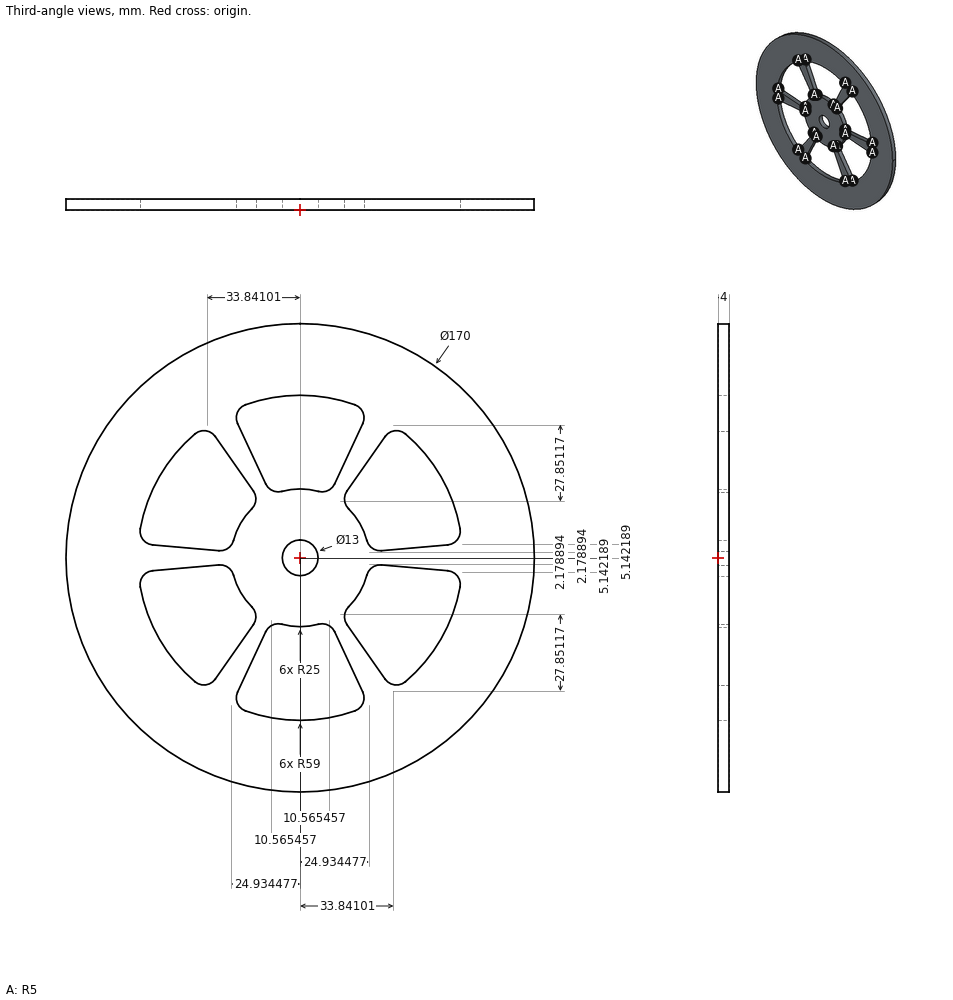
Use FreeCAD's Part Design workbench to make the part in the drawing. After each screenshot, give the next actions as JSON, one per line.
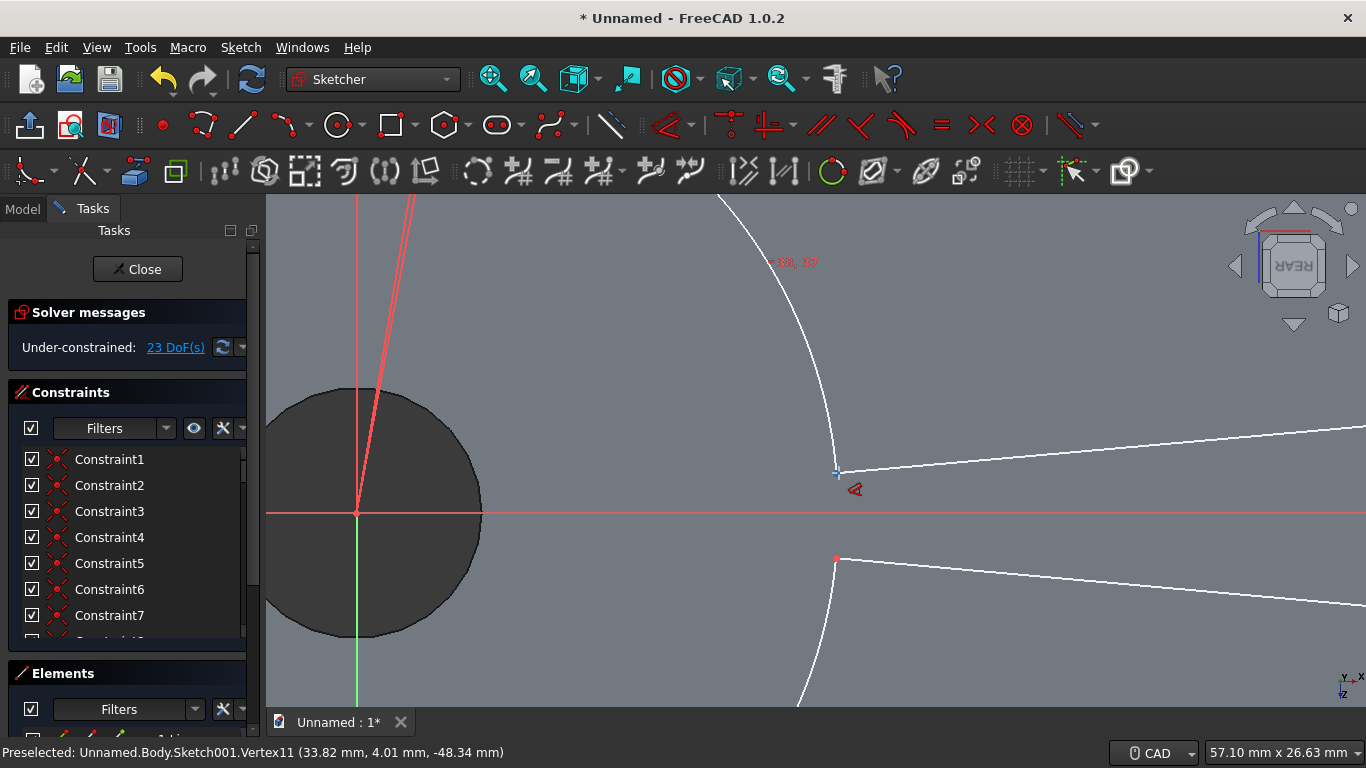
{"action": "left_click", "coordinate": [837, 473]}
{"action": "left_click", "coordinate": [871, 493]}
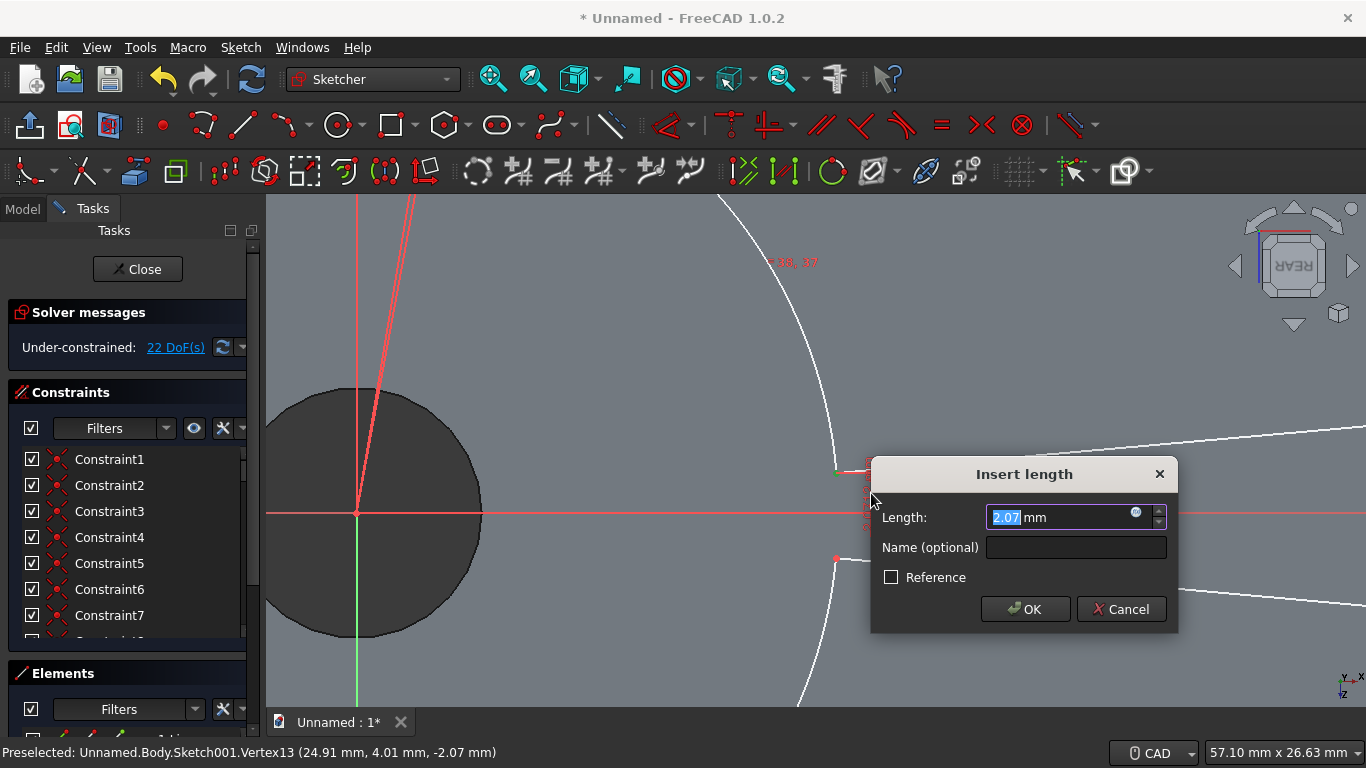
{"action": "type", "text": "2.178894"}
{"action": "key", "text": "Return"}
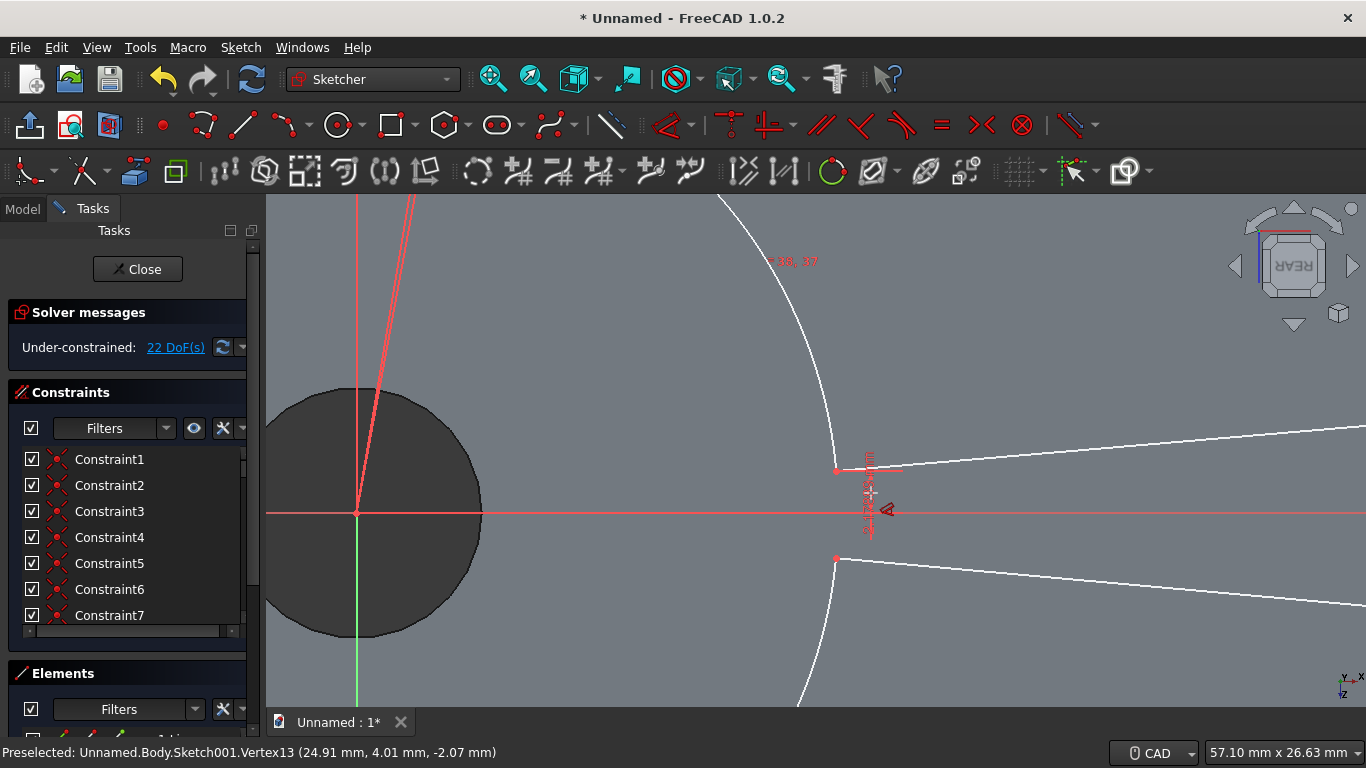
{"action": "scroll", "coordinate": [809, 441], "scroll_direction": "down", "scroll_amount": 10}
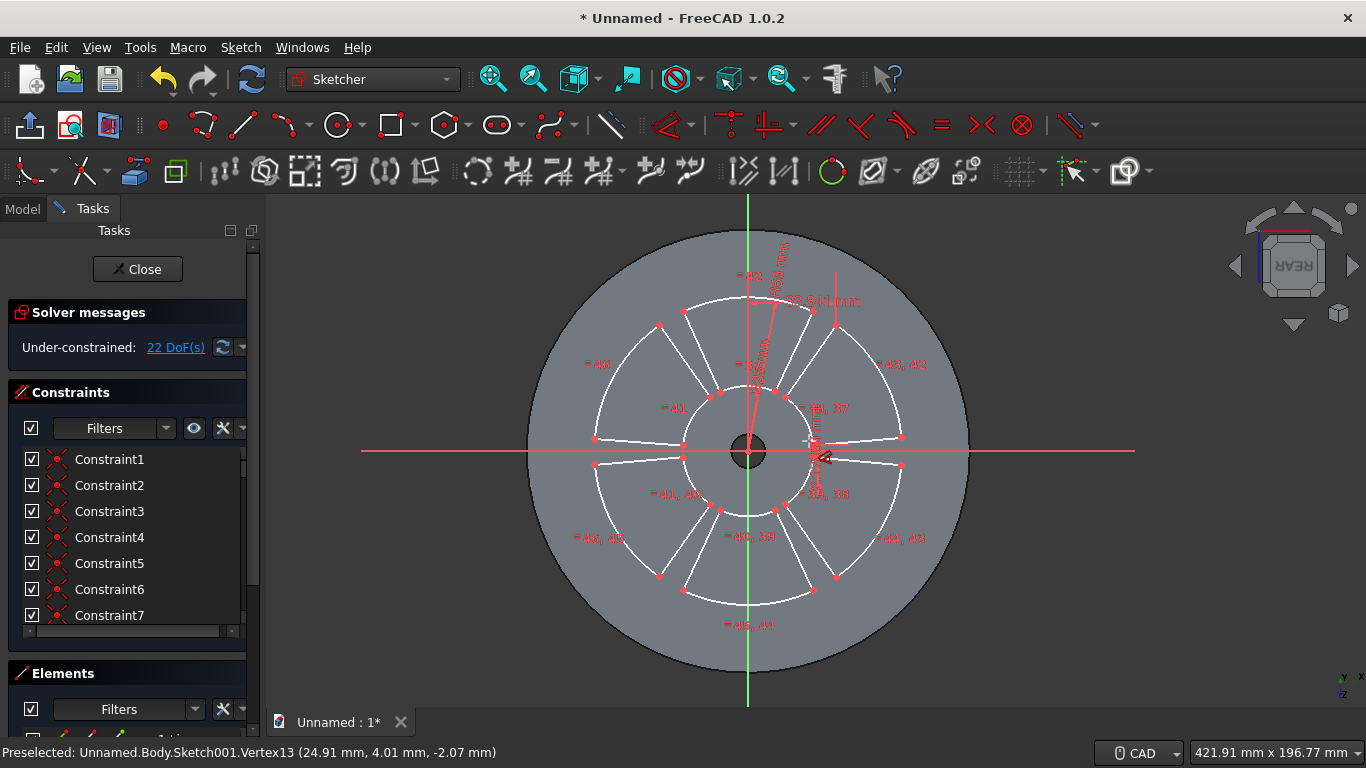
{"action": "scroll", "coordinate": [901, 438], "scroll_direction": "up", "scroll_amount": 6}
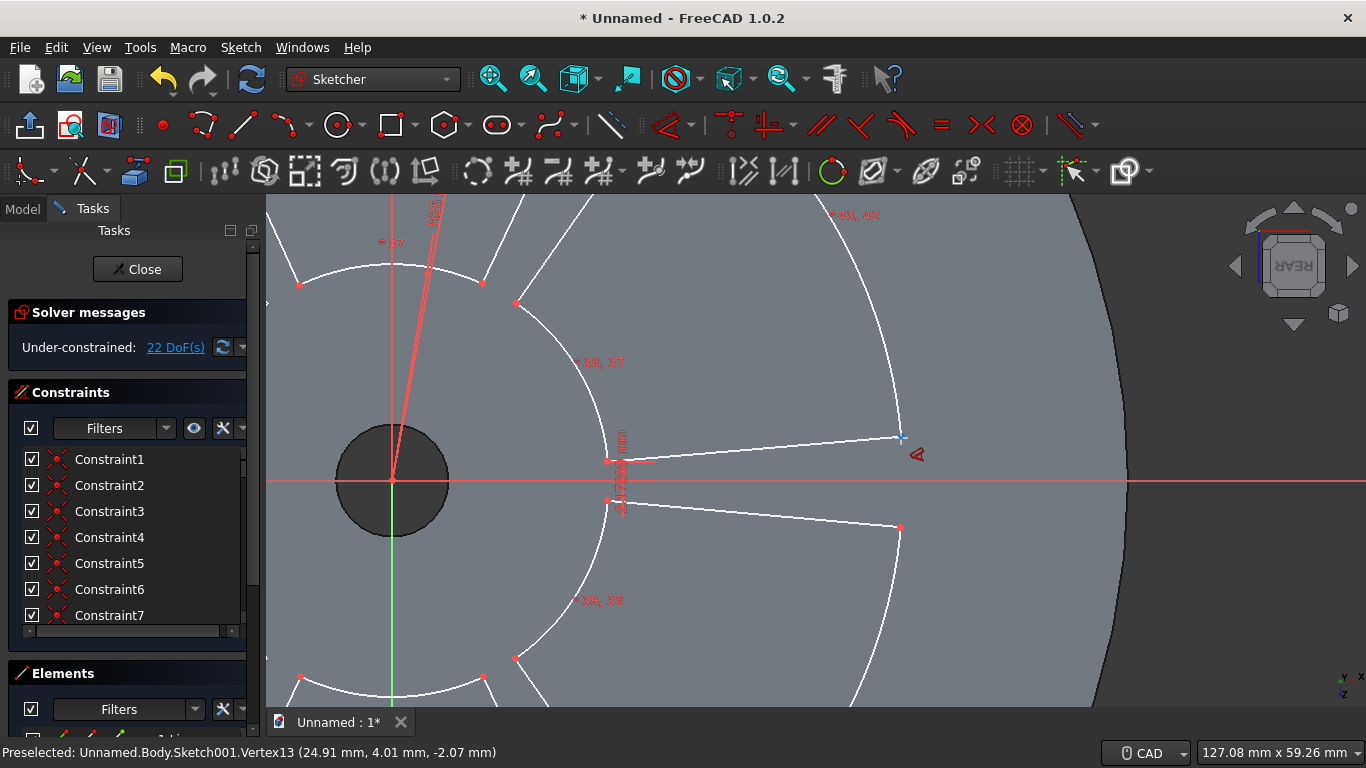
{"action": "left_click", "coordinate": [901, 437]}
{"action": "left_click", "coordinate": [935, 459]}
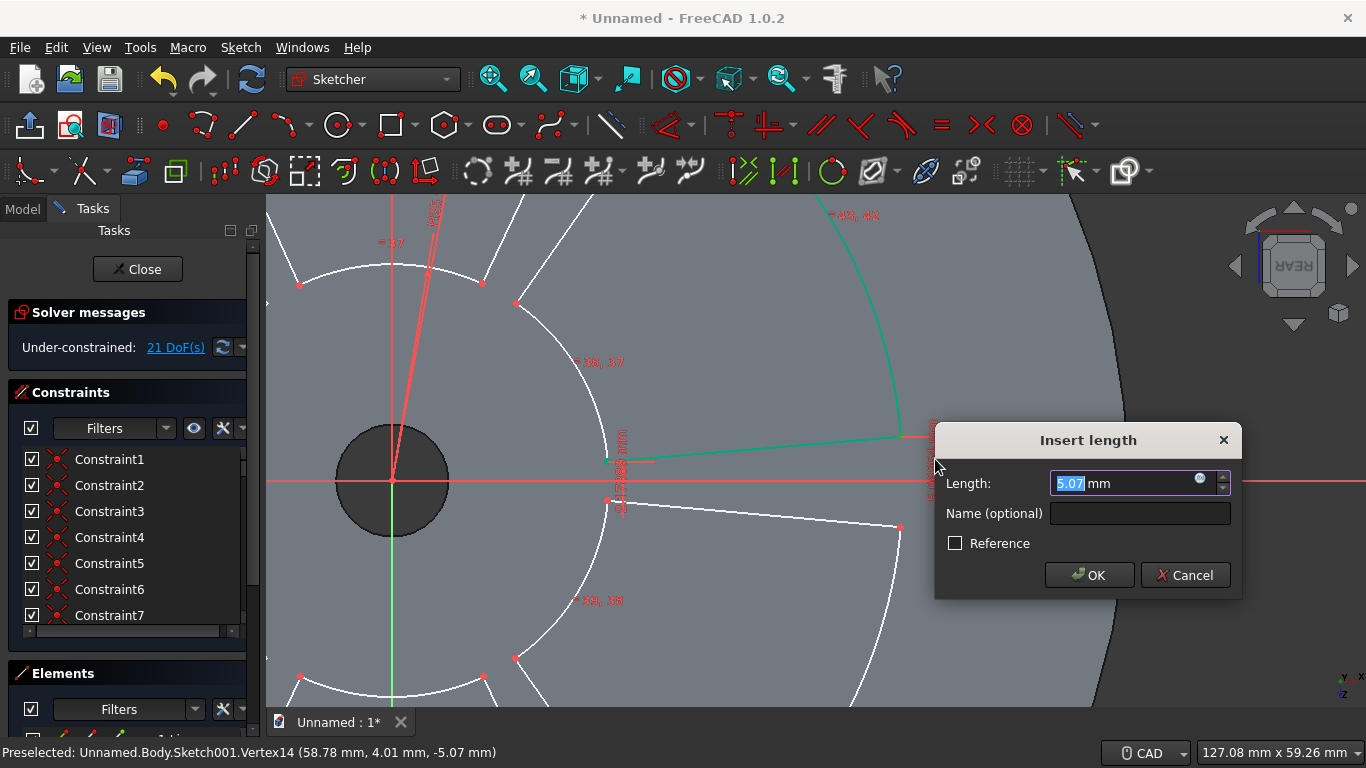
{"action": "type", "text": "5.142189"}
{"action": "key", "text": "Return"}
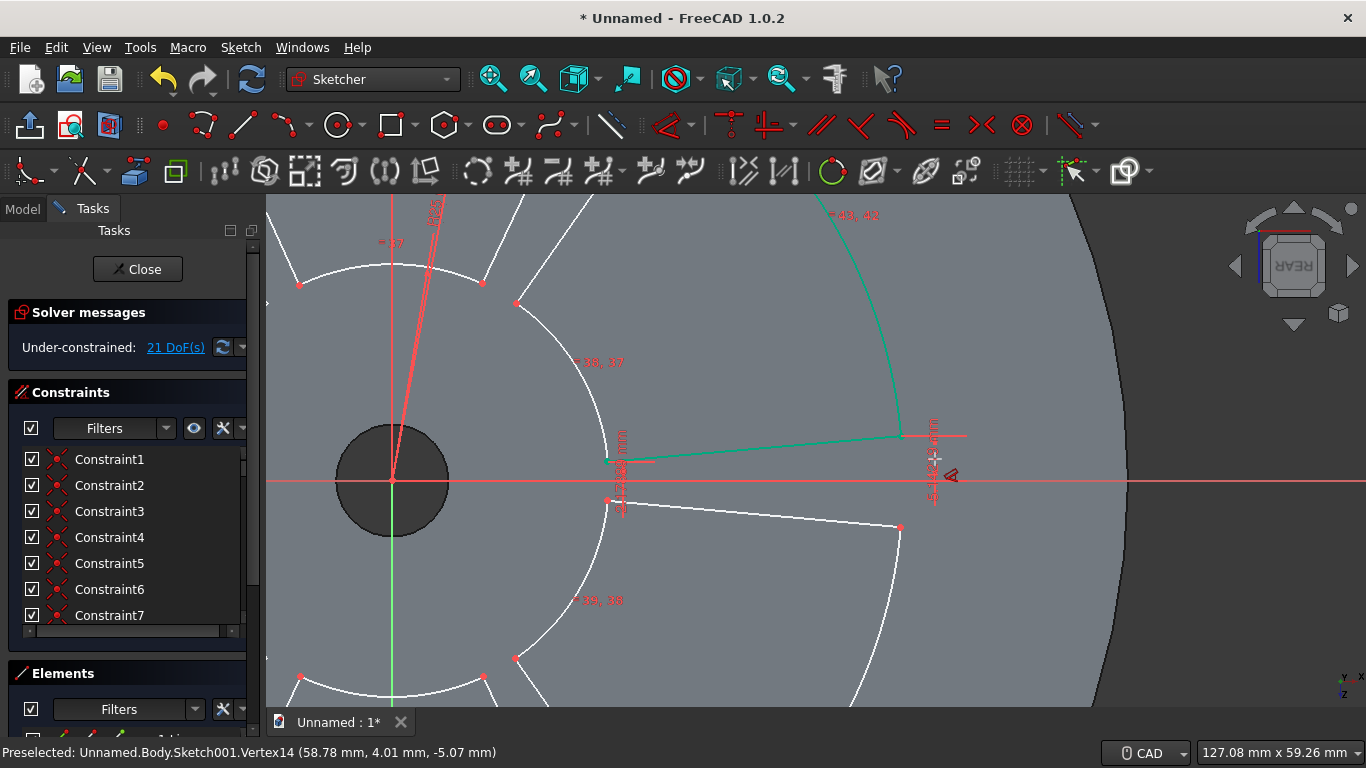
{"action": "left_click", "coordinate": [901, 527]}
{"action": "left_click", "coordinate": [935, 504]}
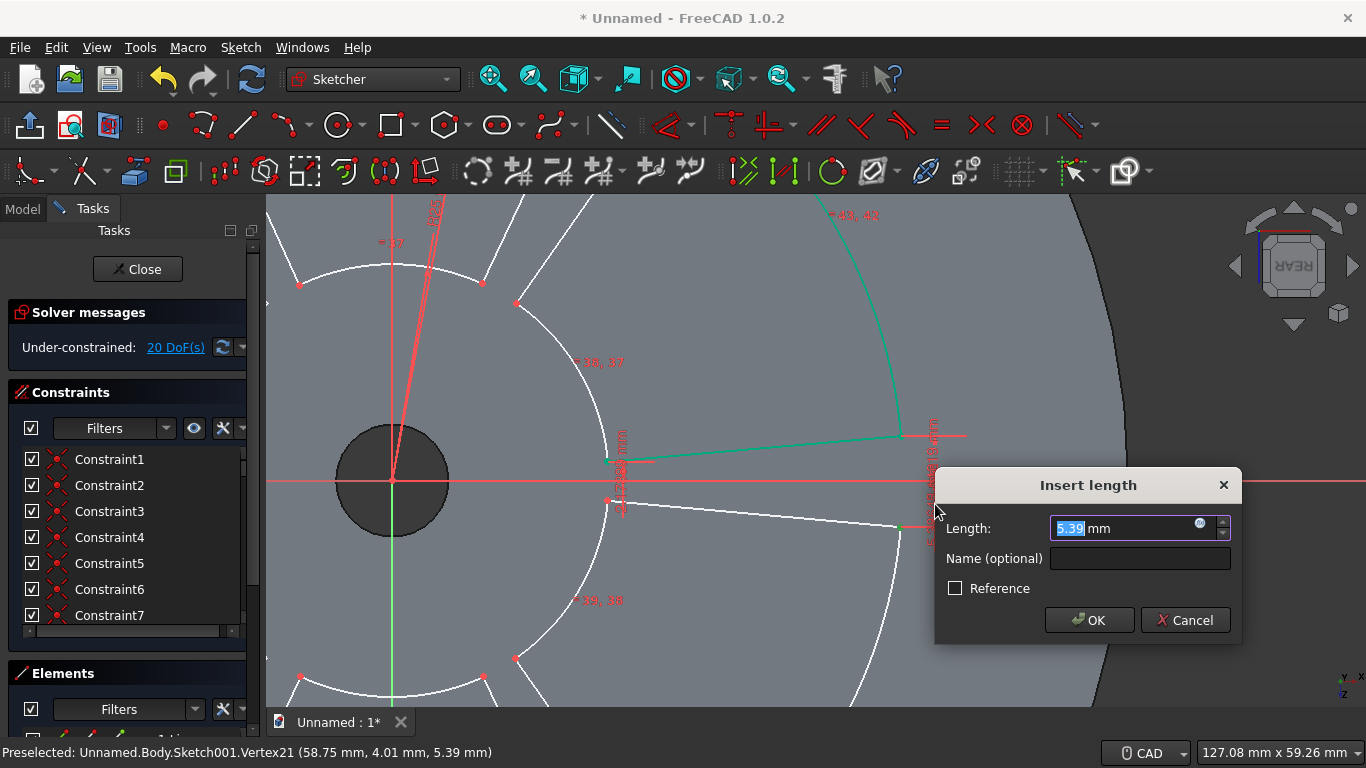
{"action": "type", "text": "5.142189"}
{"action": "key", "text": "Return"}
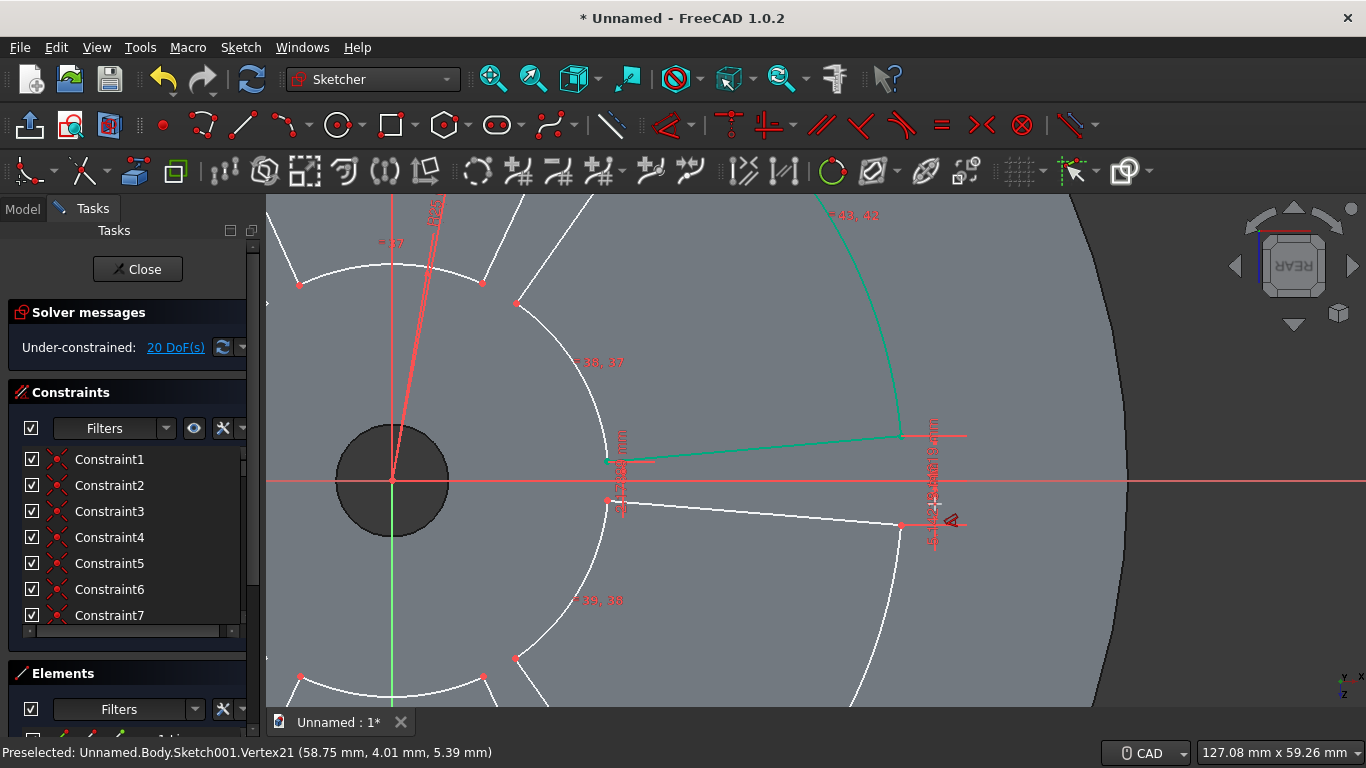
{"action": "scroll", "coordinate": [608, 501], "scroll_direction": "up", "scroll_amount": 4}